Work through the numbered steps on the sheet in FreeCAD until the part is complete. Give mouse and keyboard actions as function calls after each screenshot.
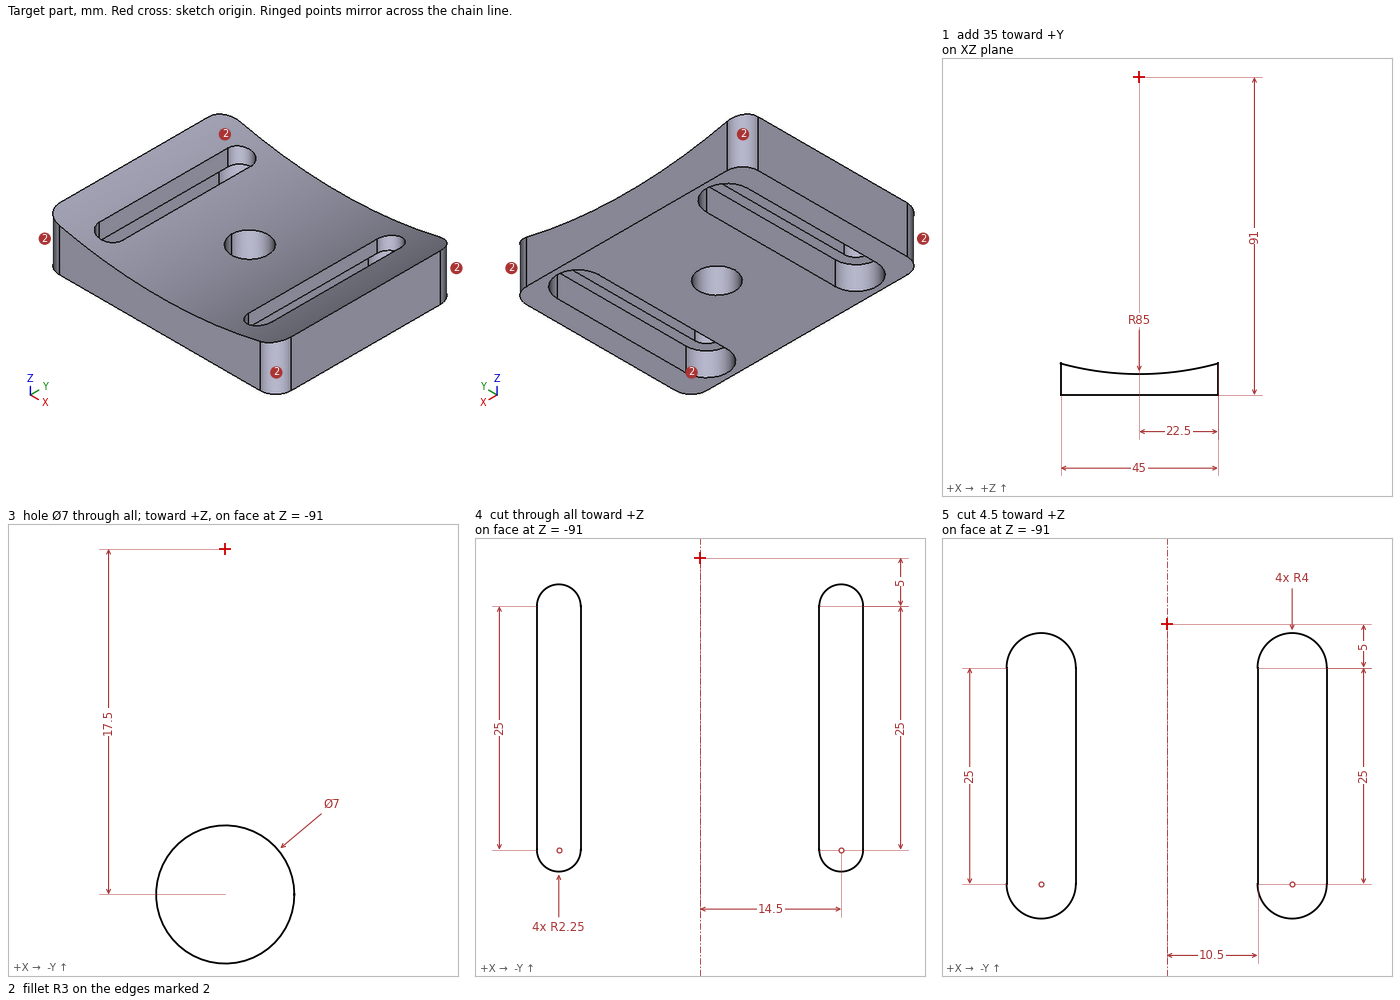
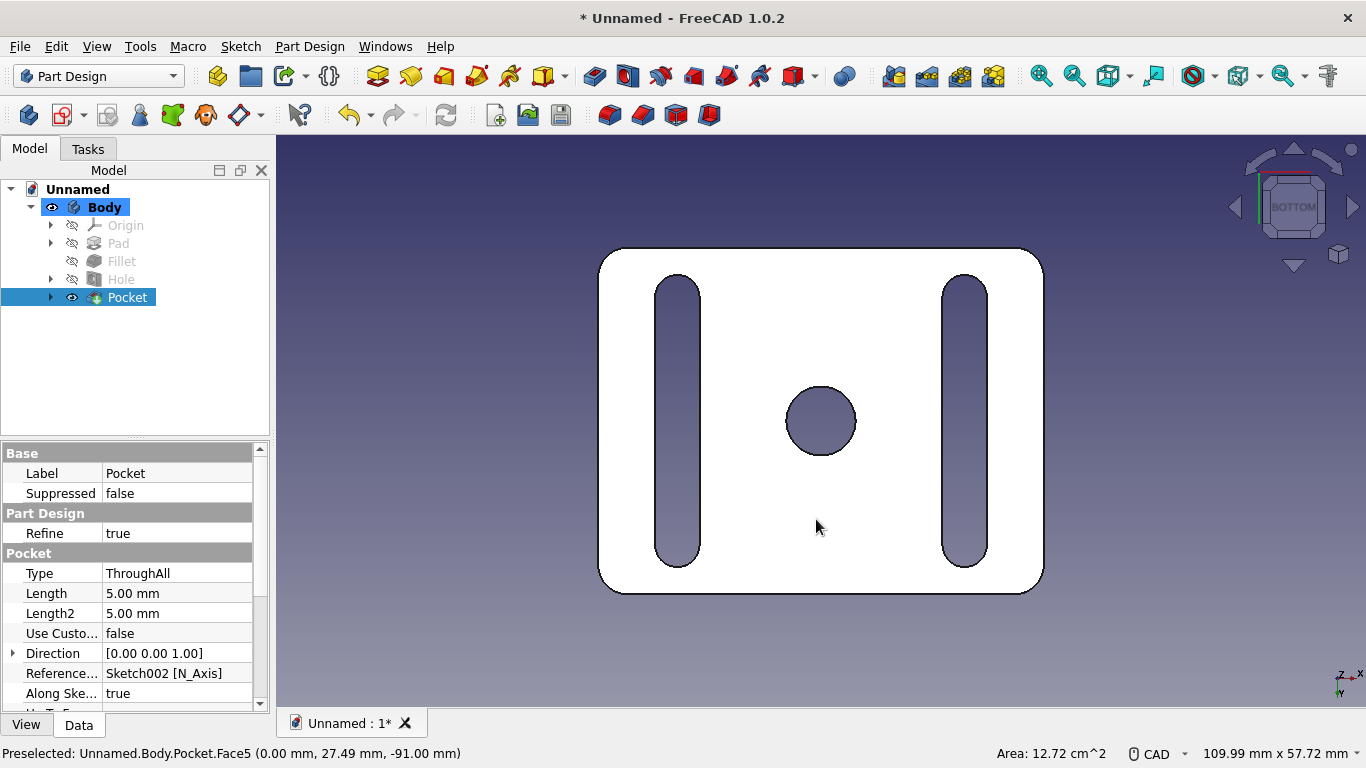
click(62, 116)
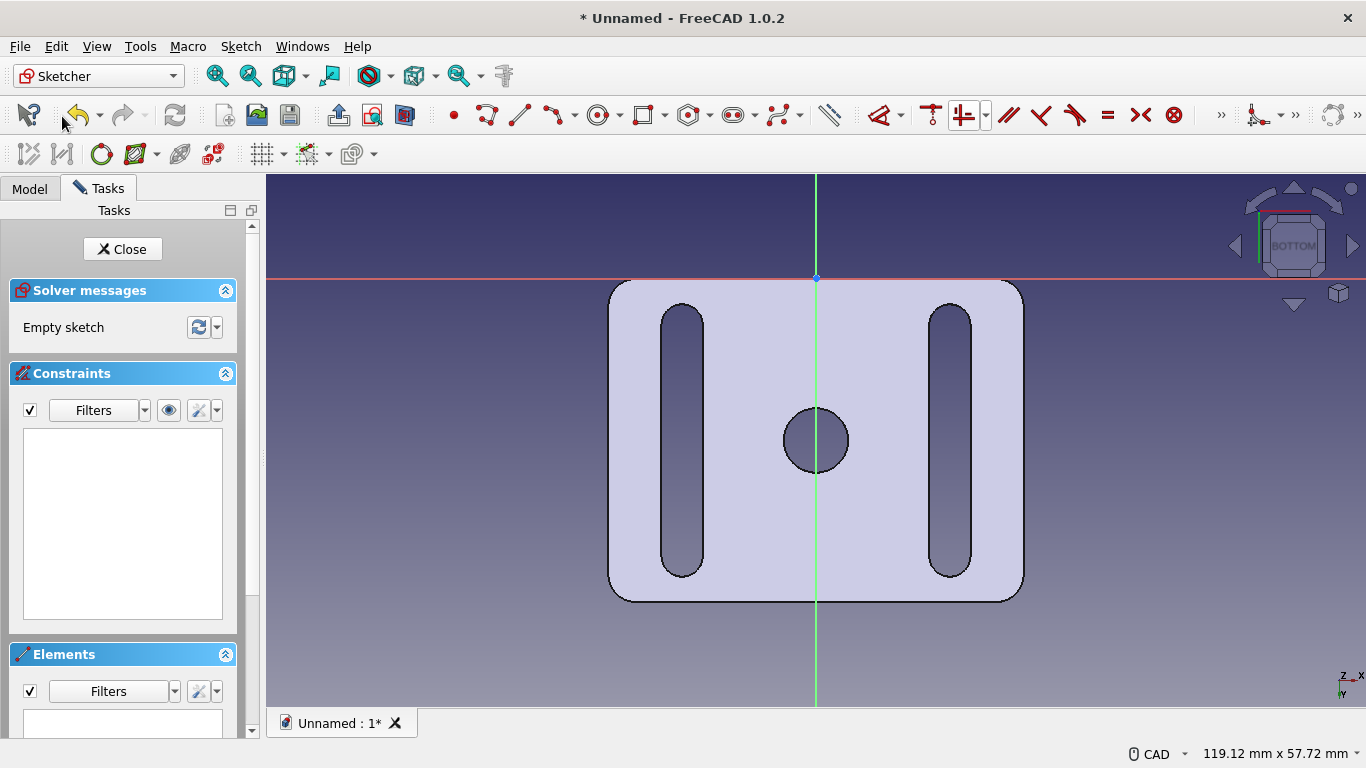
key(g)
key(s)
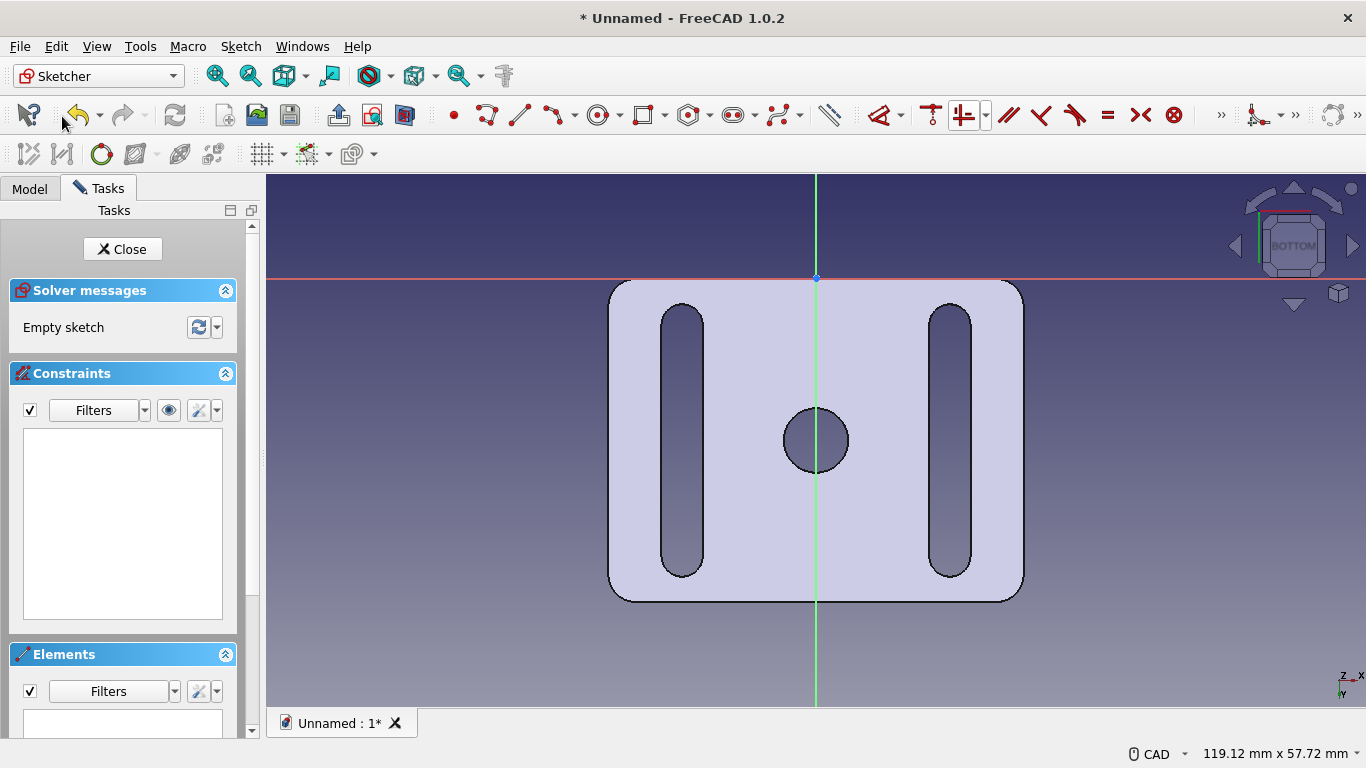
click(950, 556)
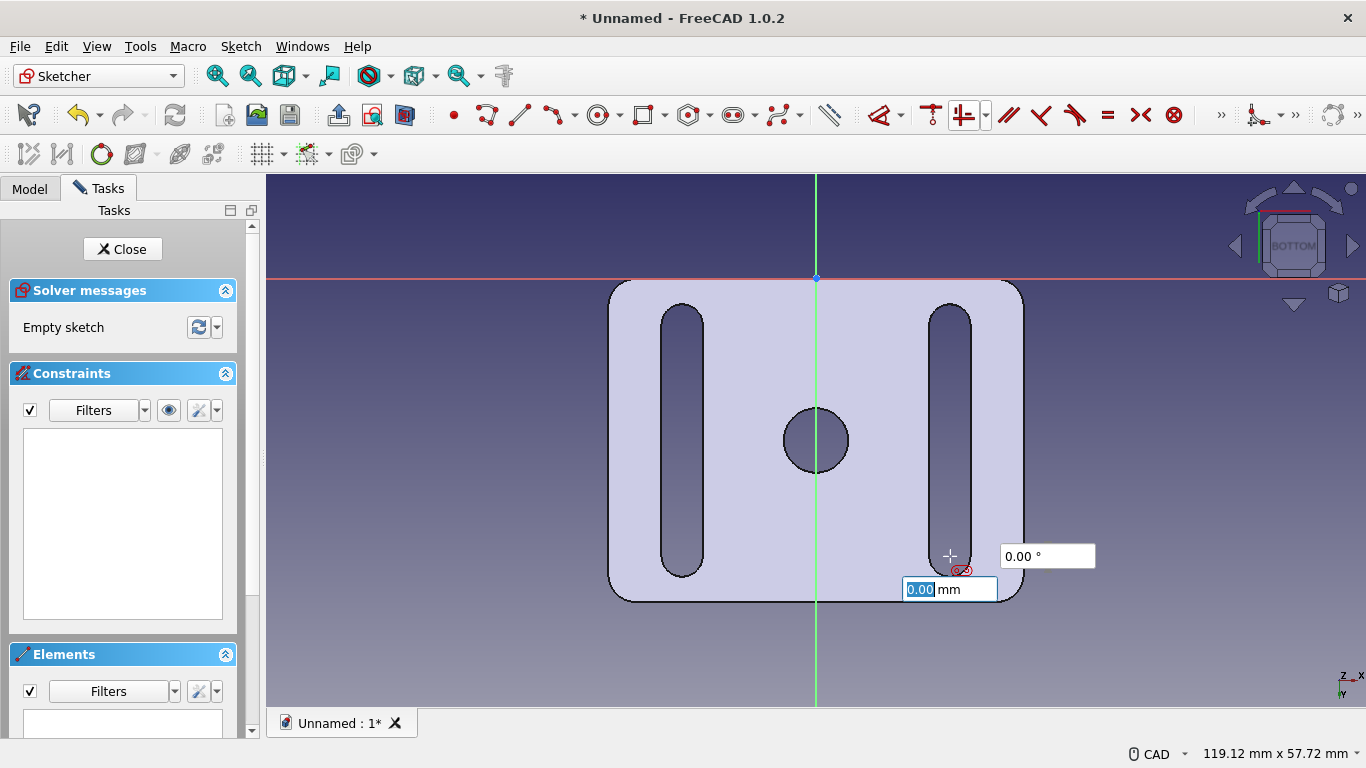
click(950, 325)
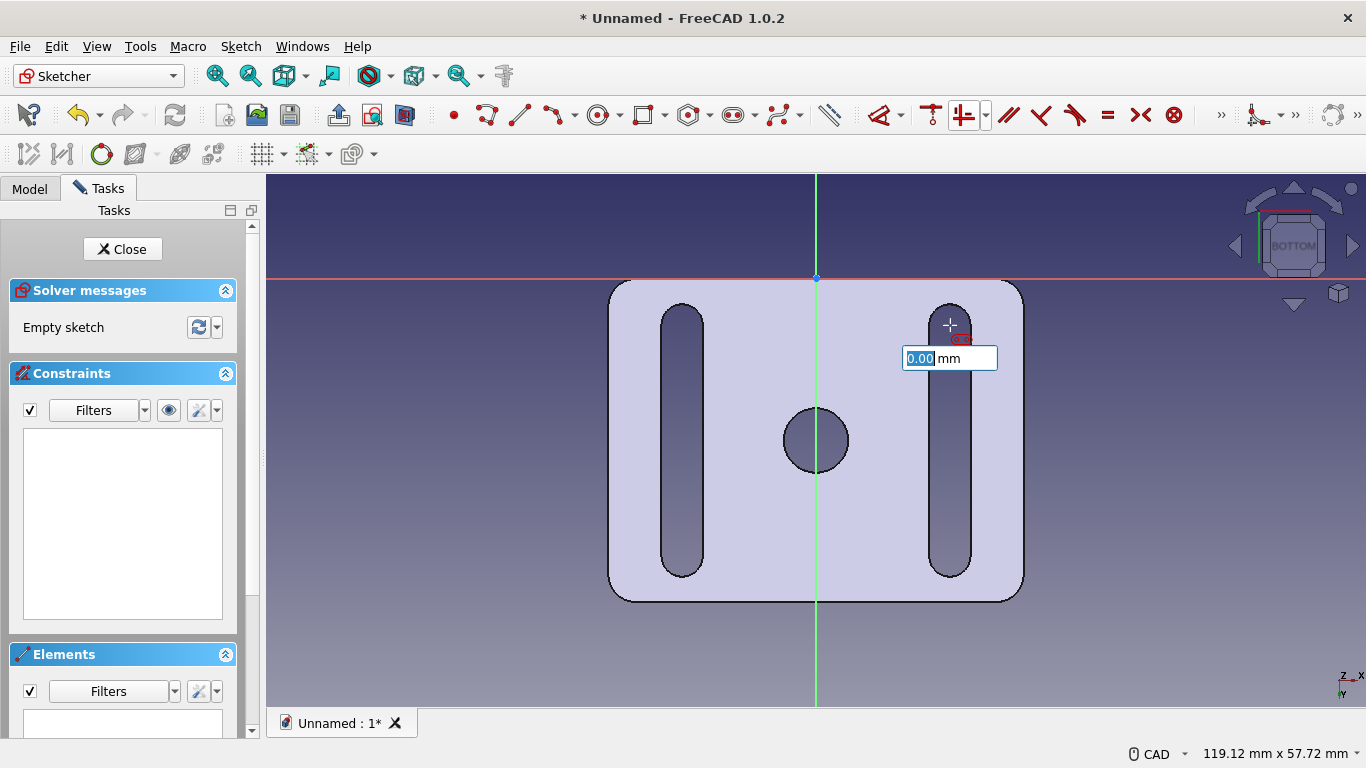
click(913, 440)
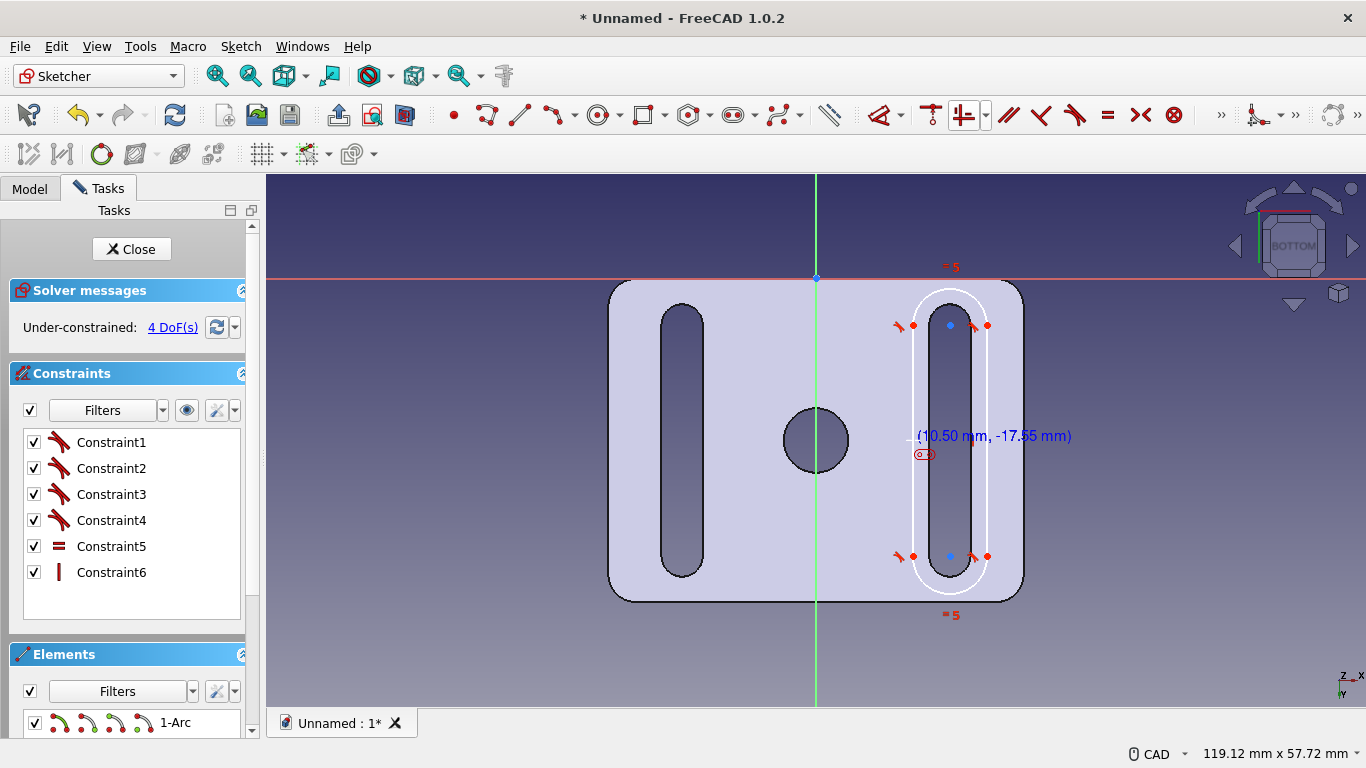
click(682, 556)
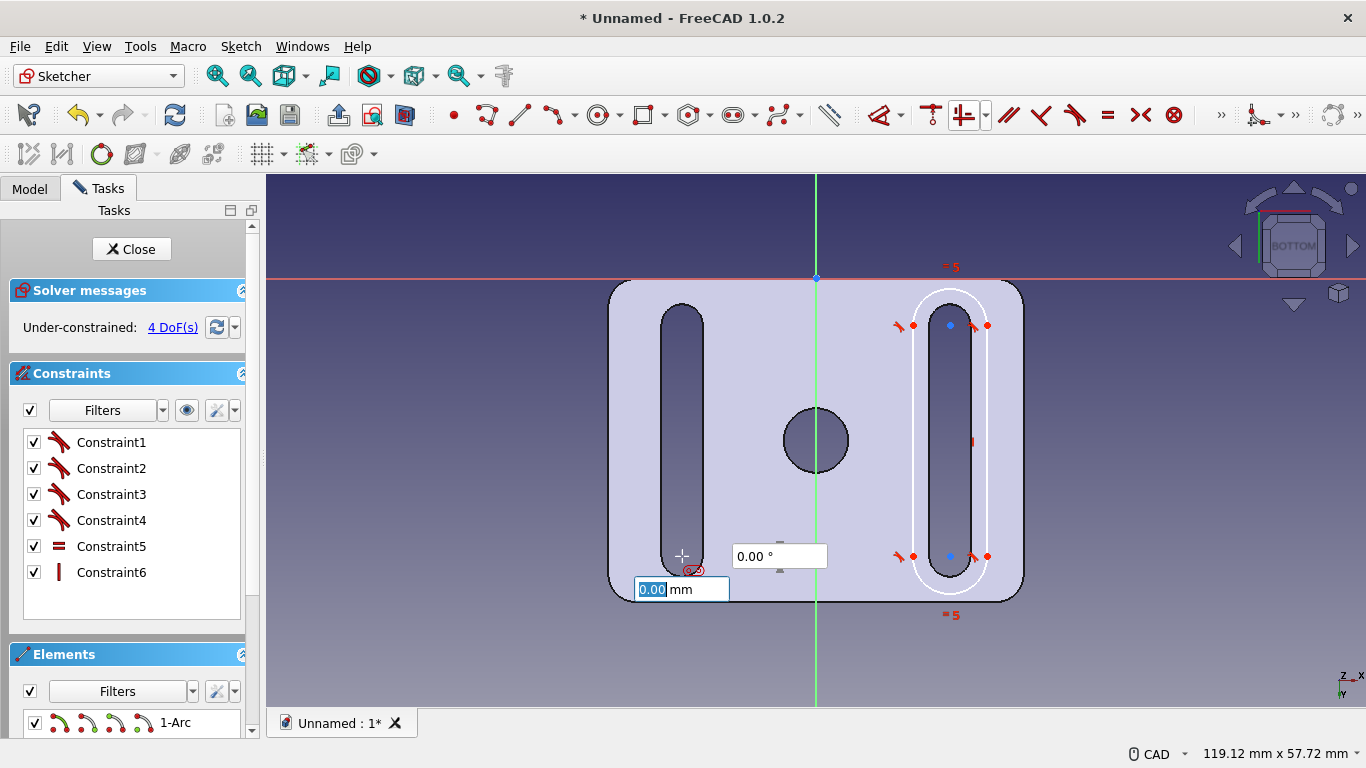
click(682, 325)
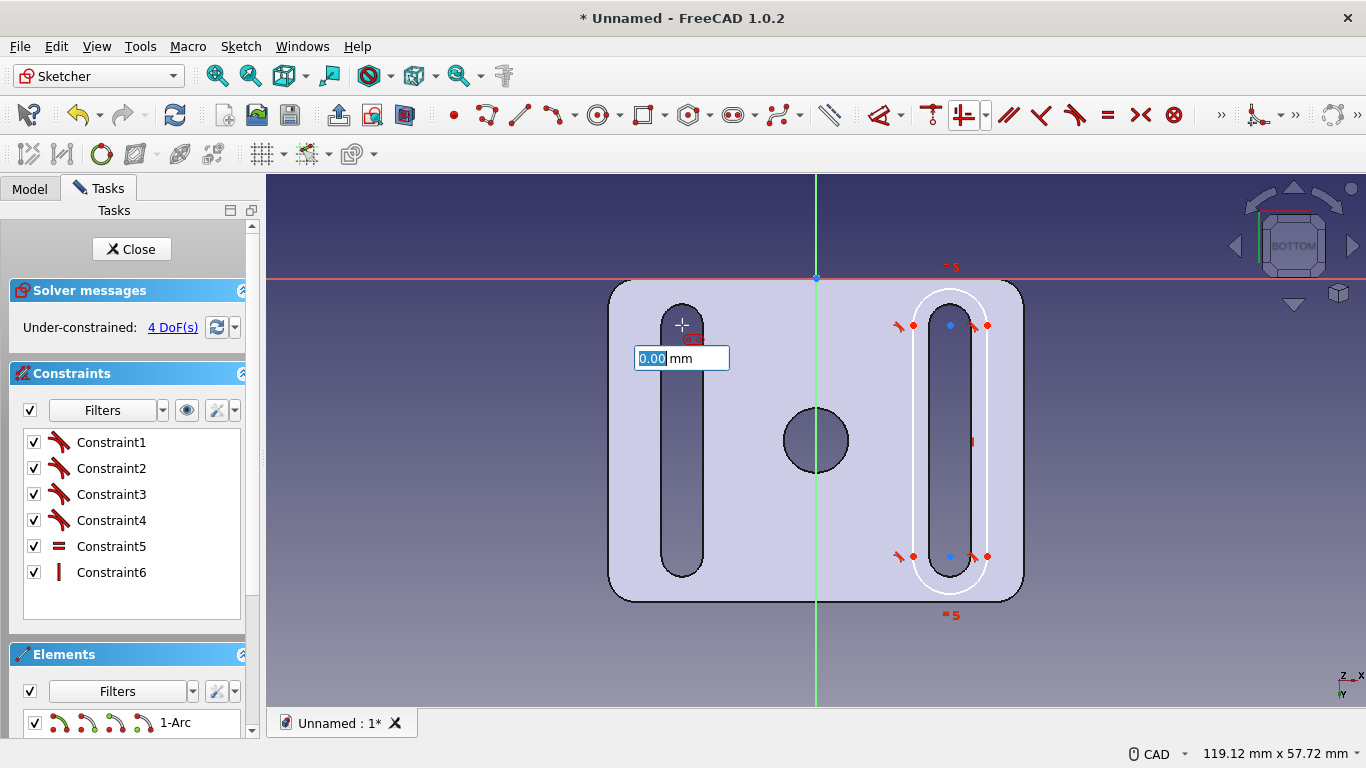
click(645, 440)
key(Escape)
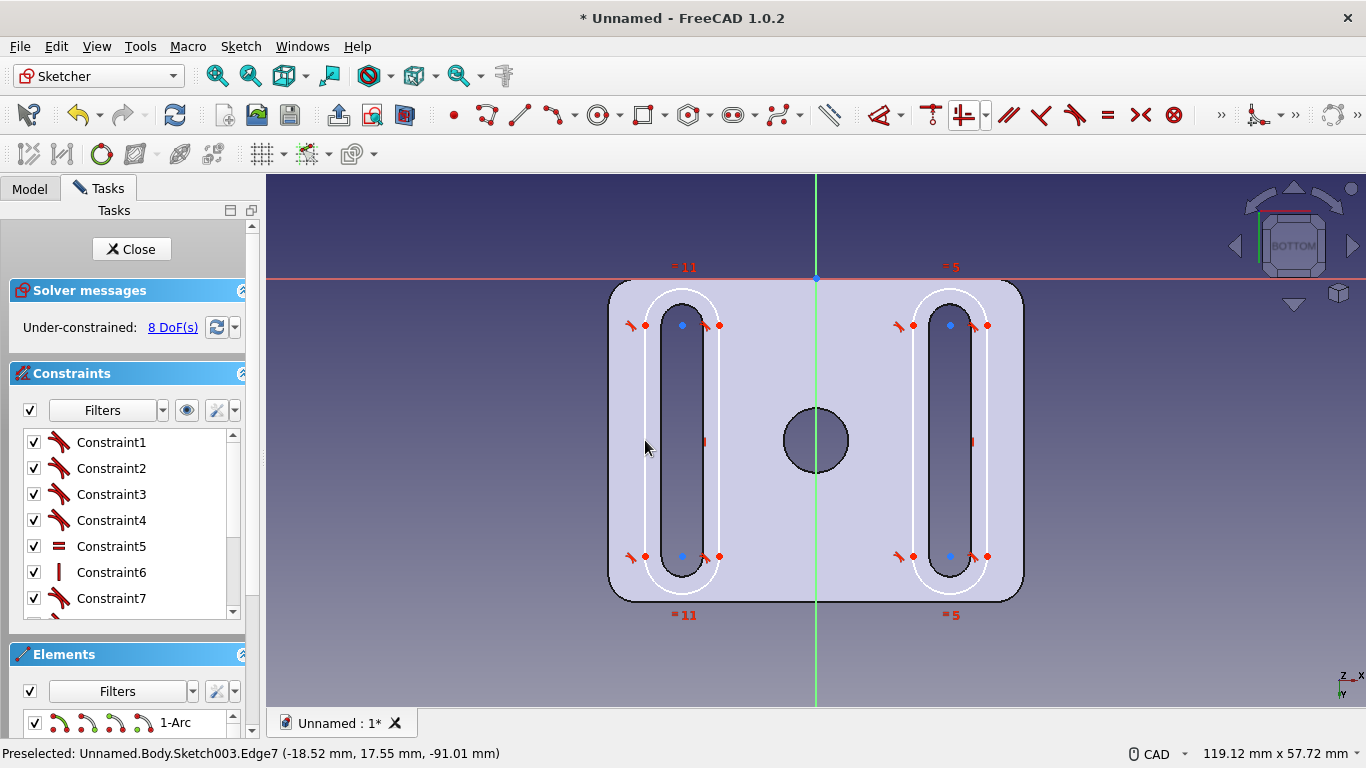
click(928, 587)